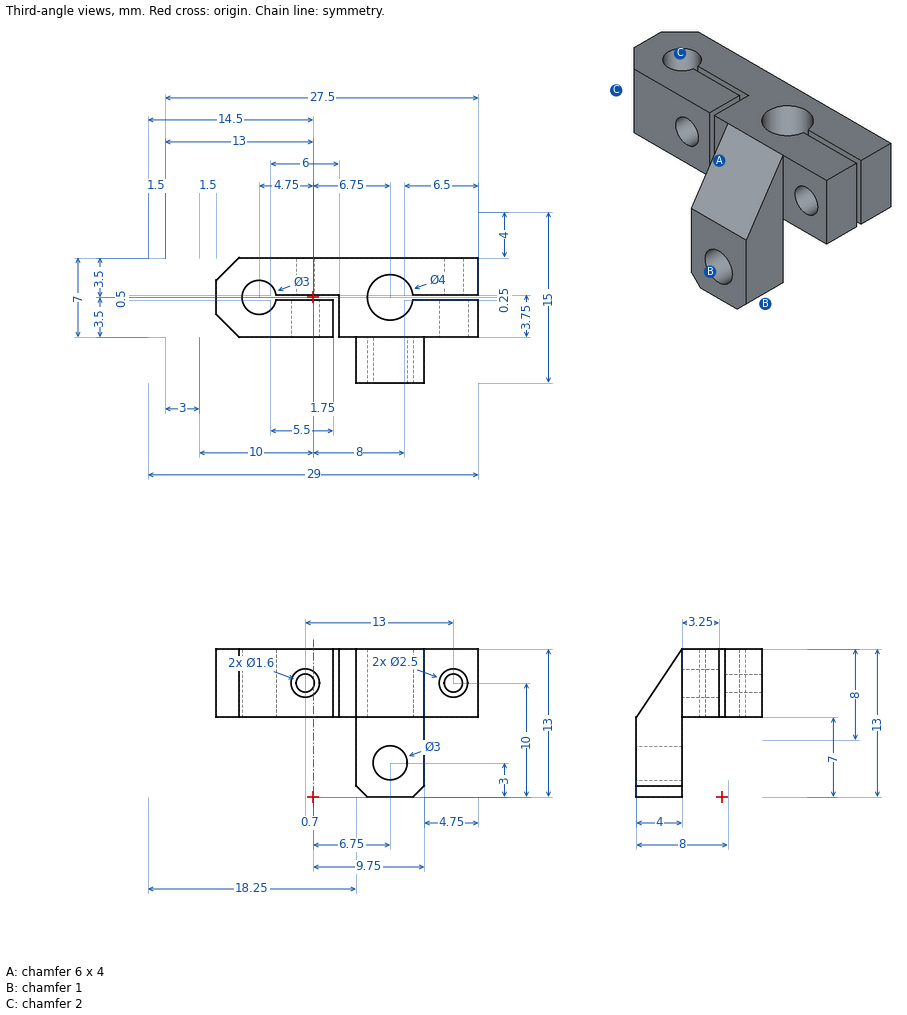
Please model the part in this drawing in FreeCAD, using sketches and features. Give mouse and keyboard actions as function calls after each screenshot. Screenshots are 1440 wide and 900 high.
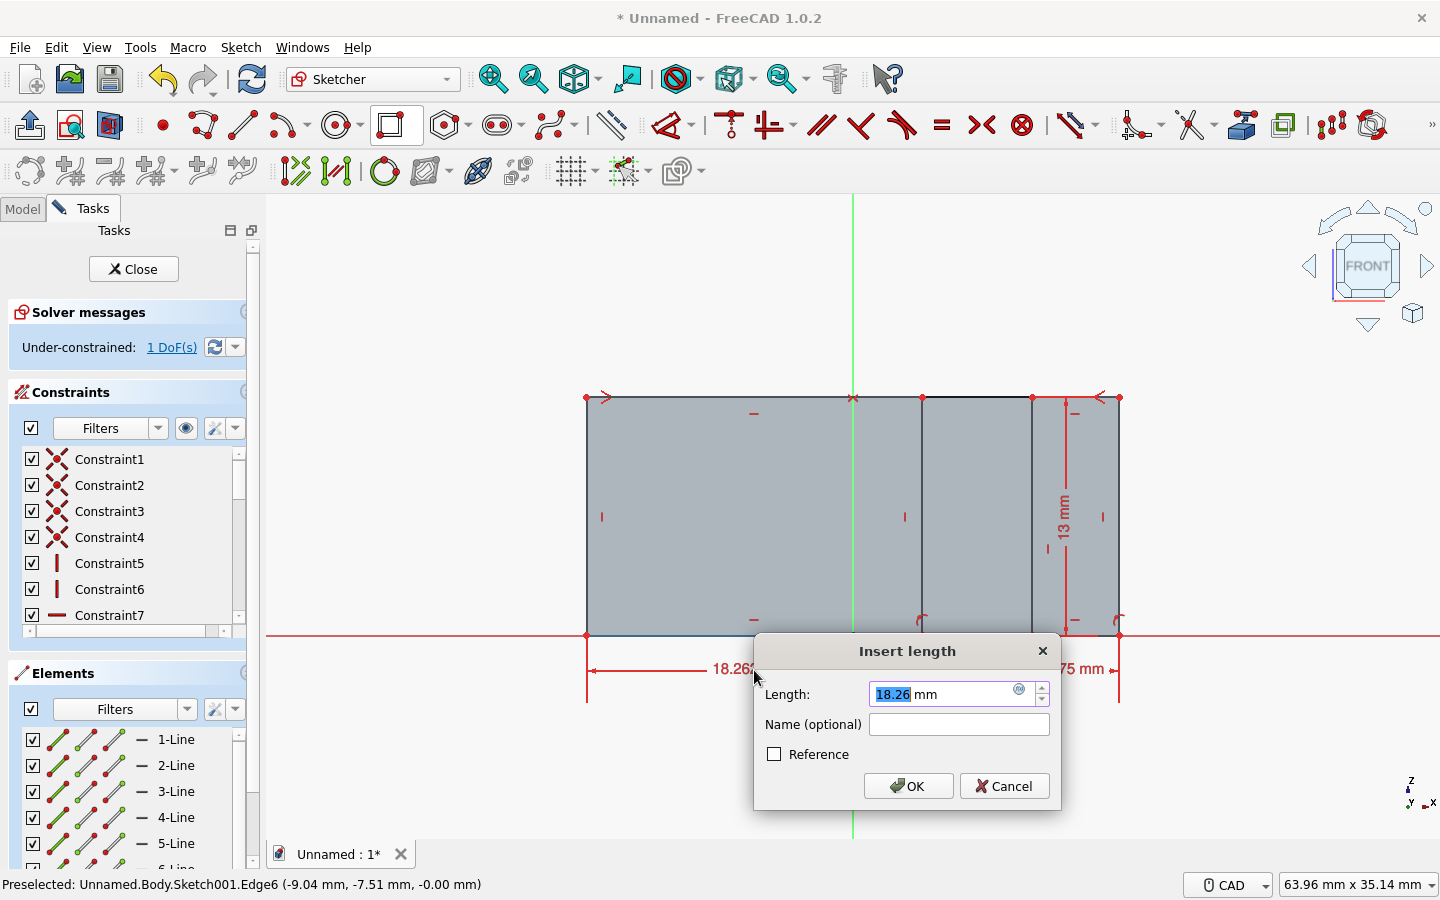
text(18.25)
key(Return)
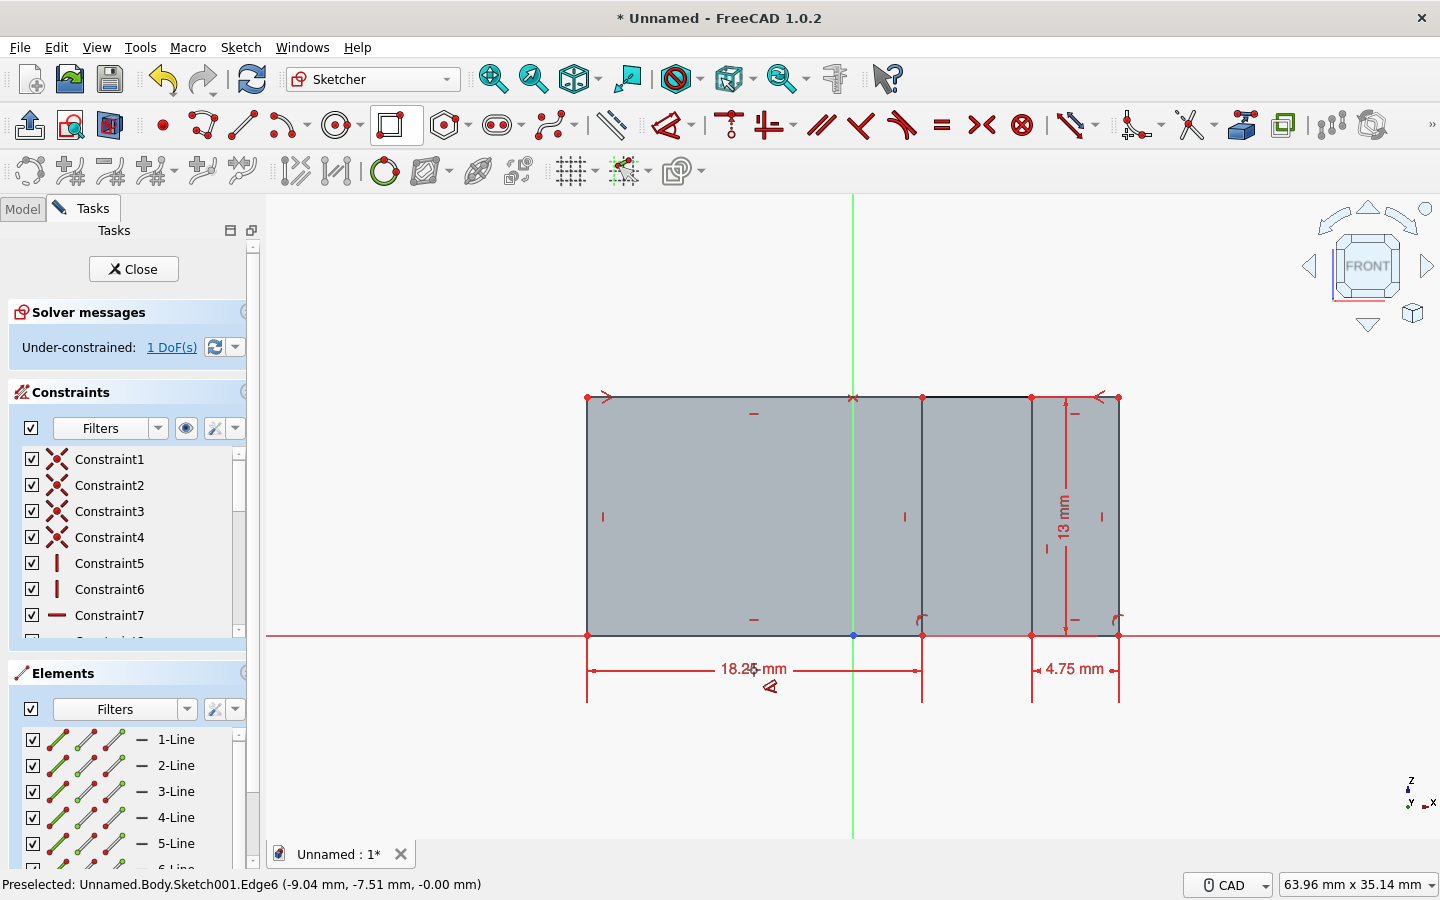
click(1032, 397)
click(942, 670)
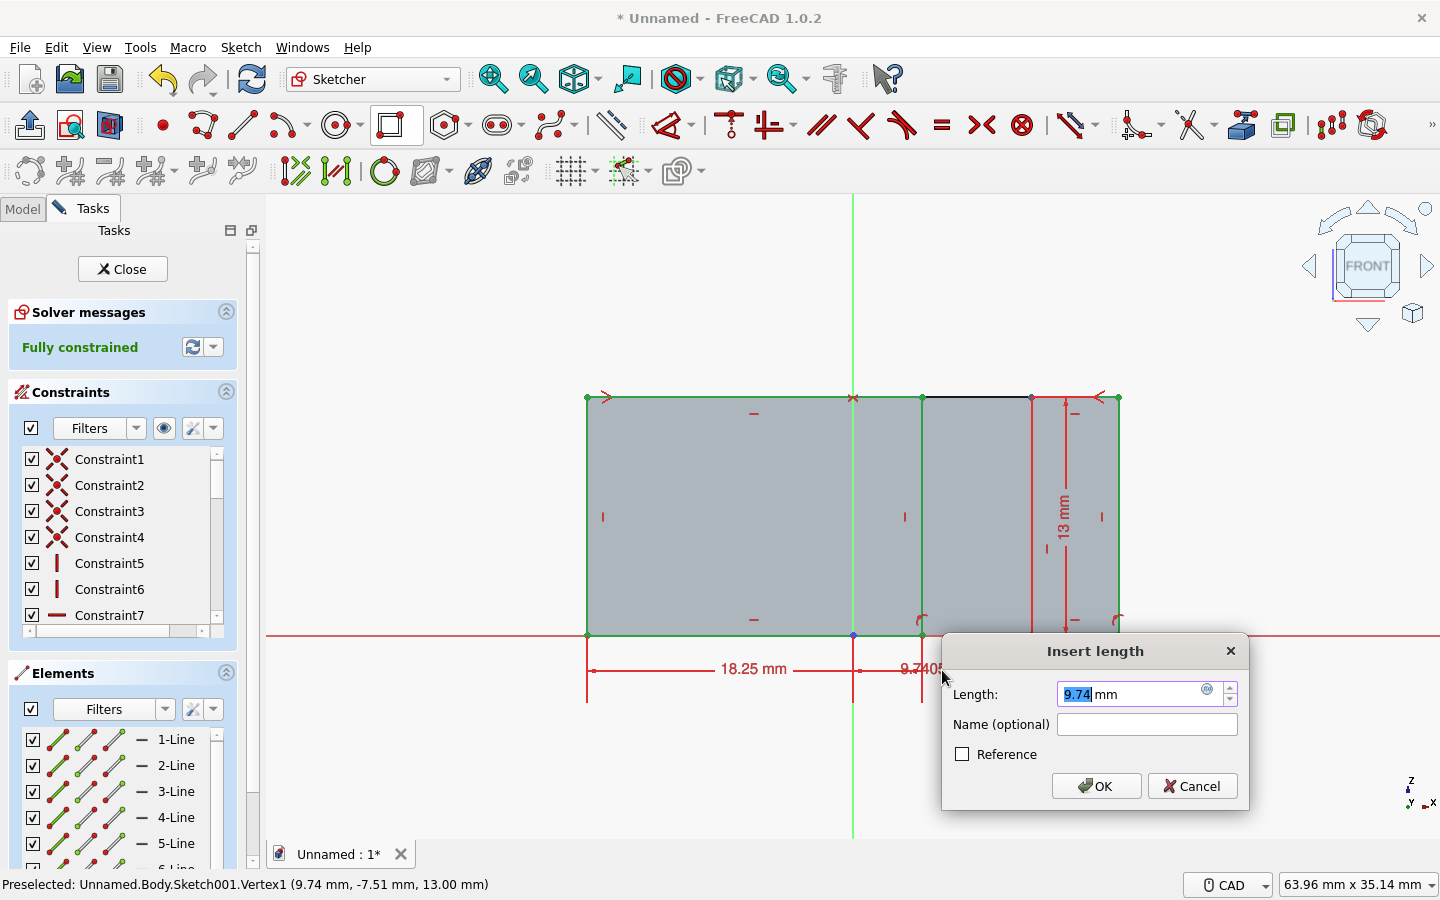
text(9.75)
key(Return)
key(Escape)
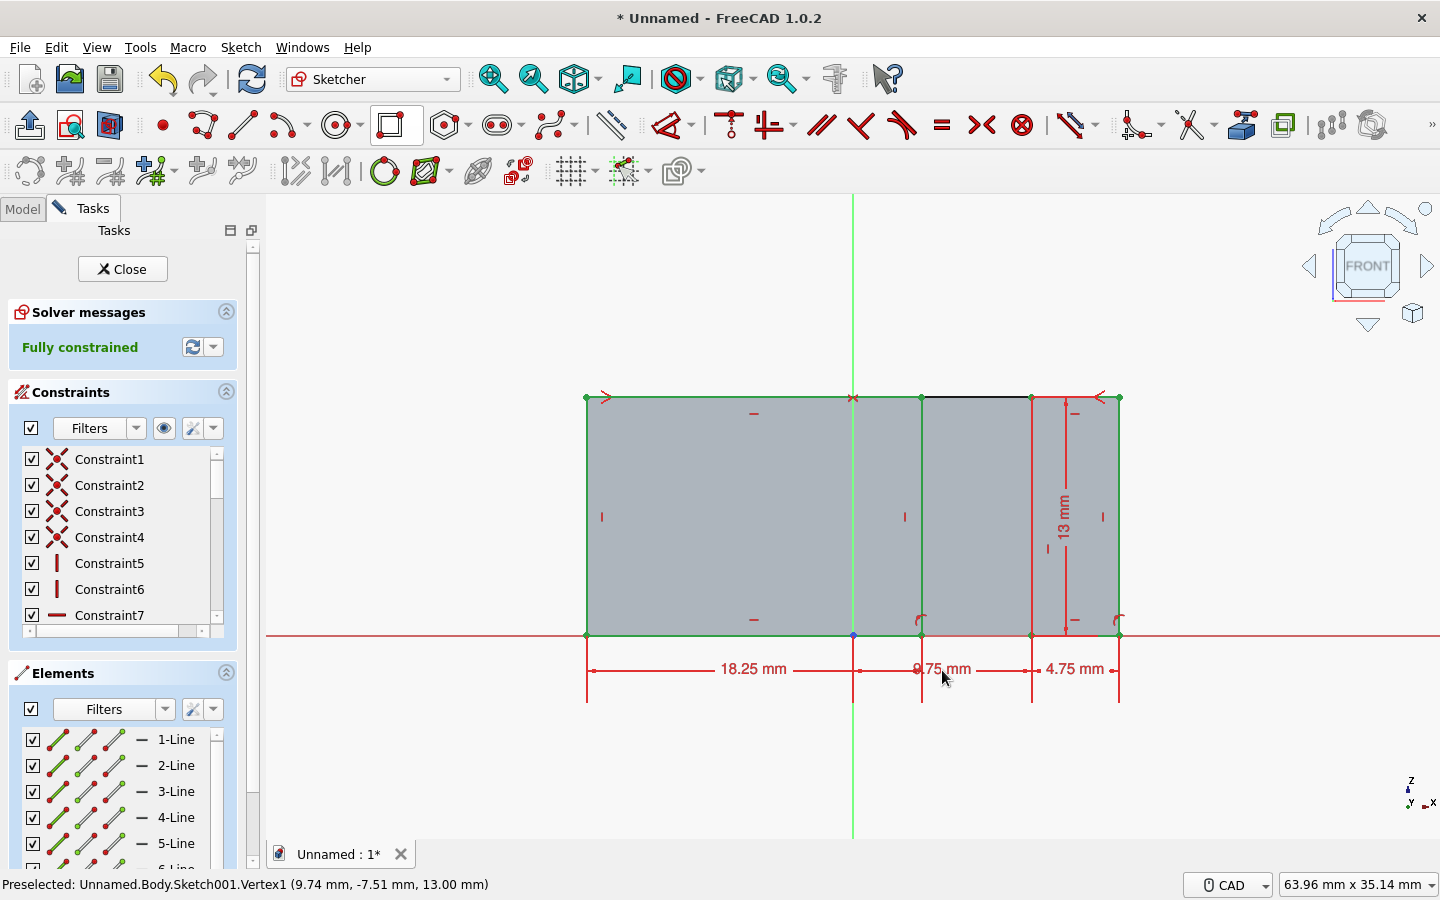
click(123, 269)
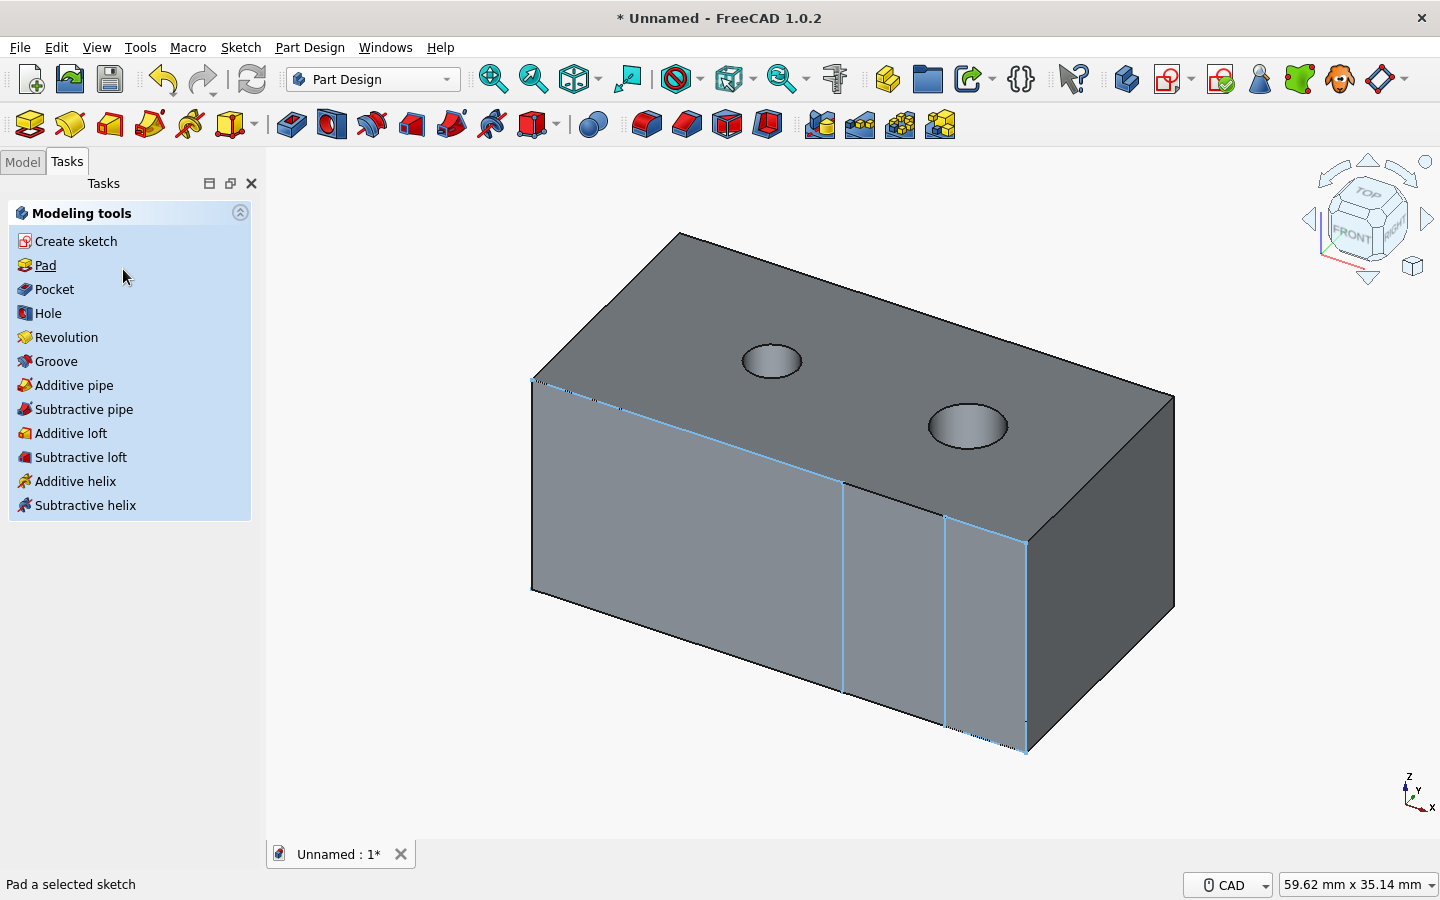
click(292, 124)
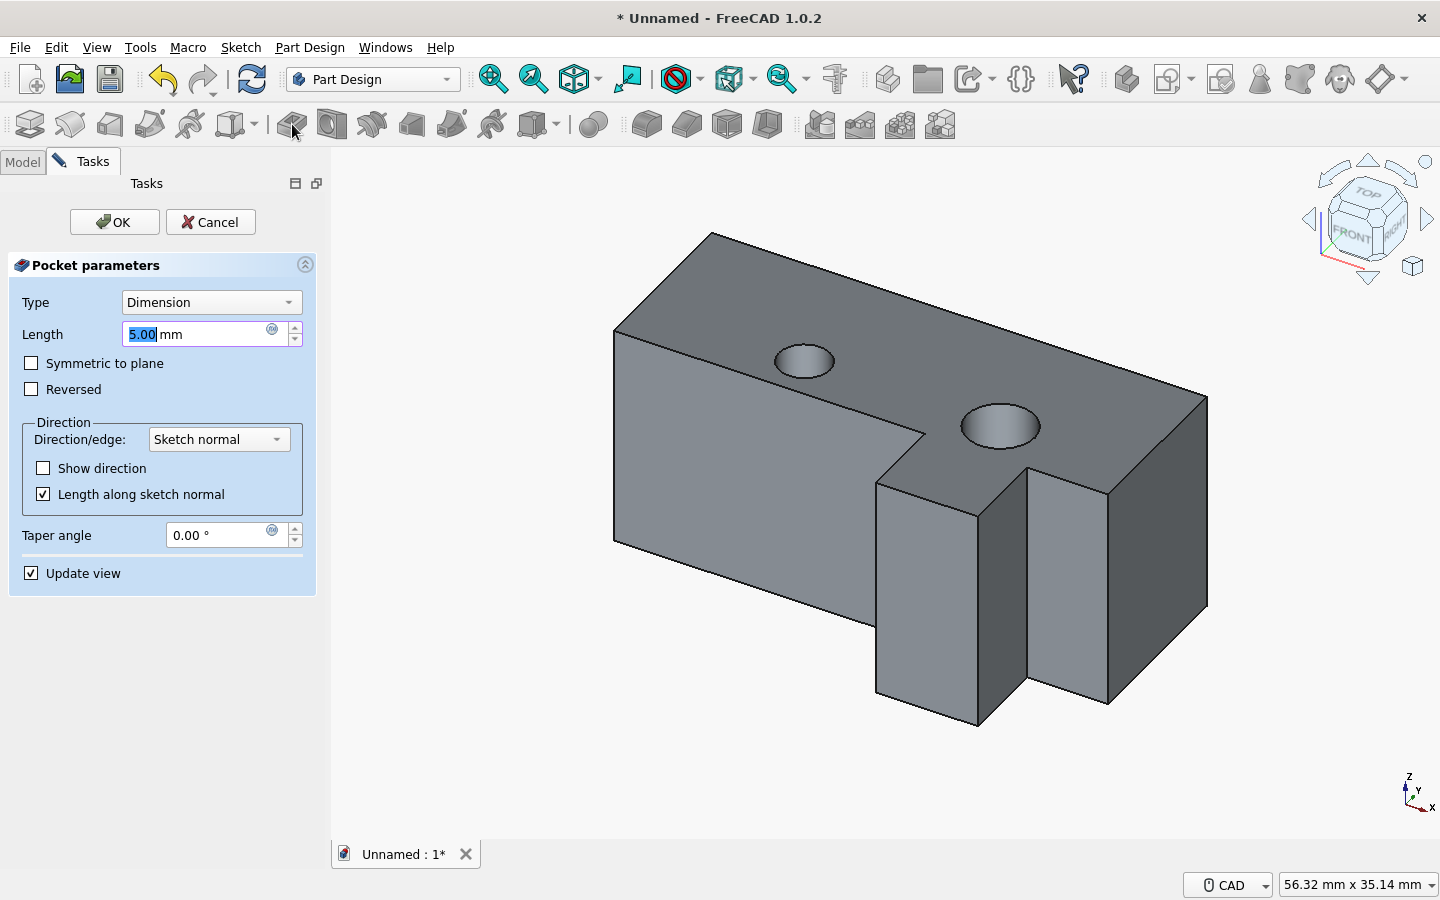
text(4)
key(Tab)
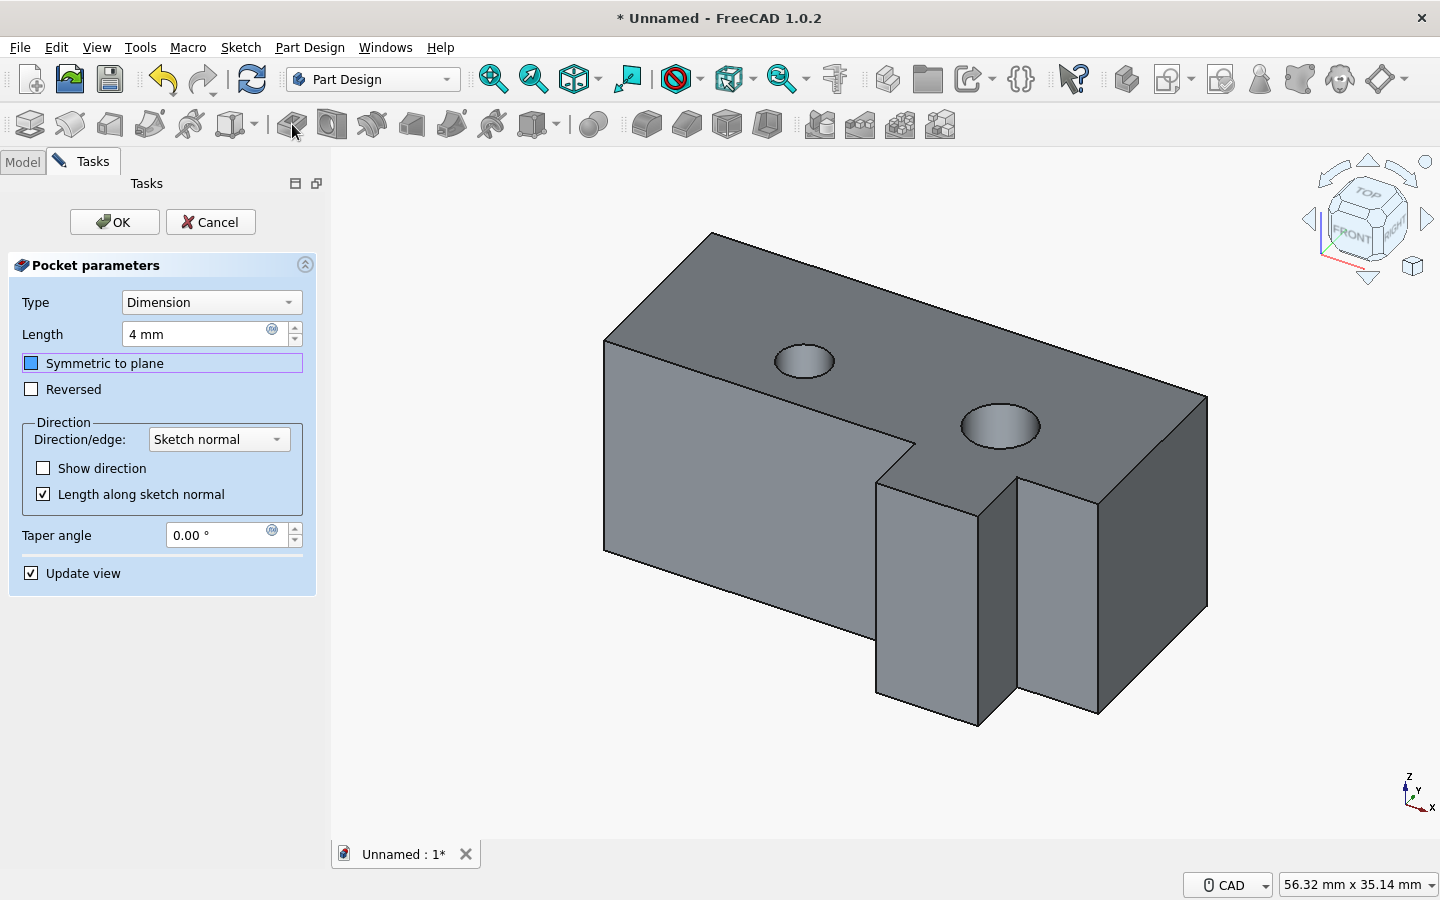
click(115, 222)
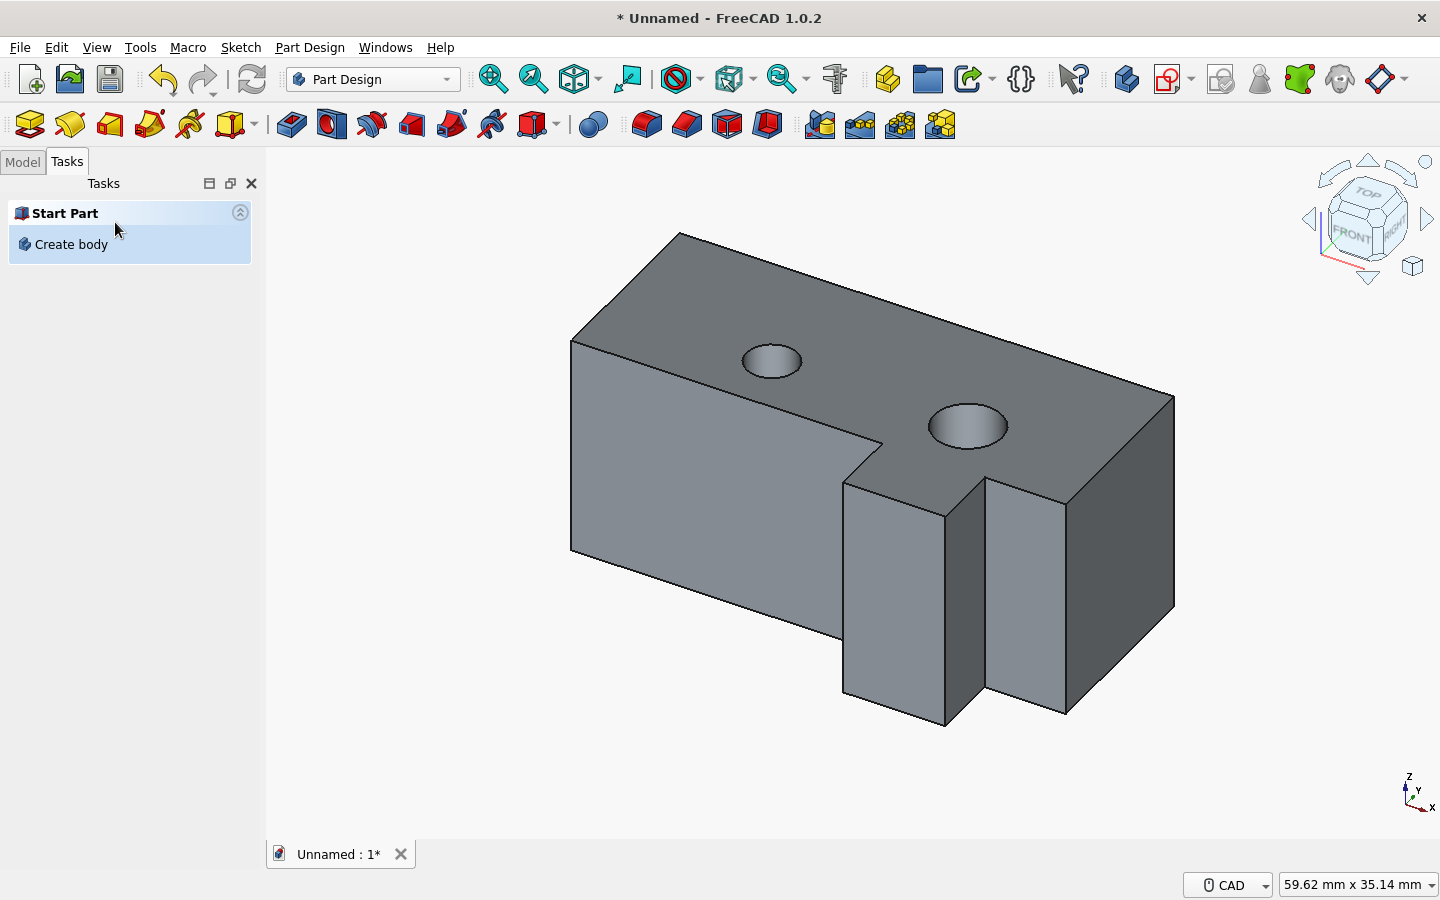
key(5)